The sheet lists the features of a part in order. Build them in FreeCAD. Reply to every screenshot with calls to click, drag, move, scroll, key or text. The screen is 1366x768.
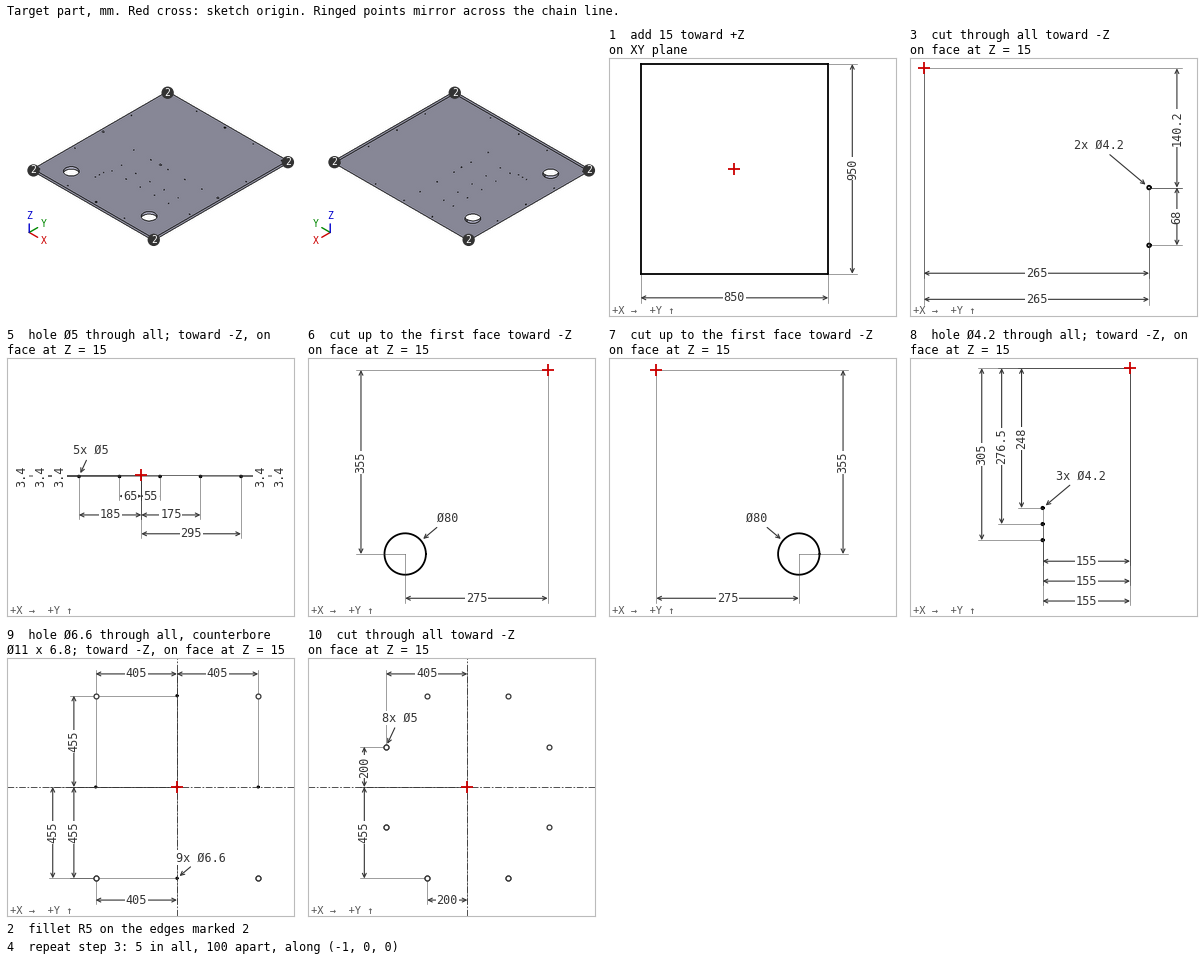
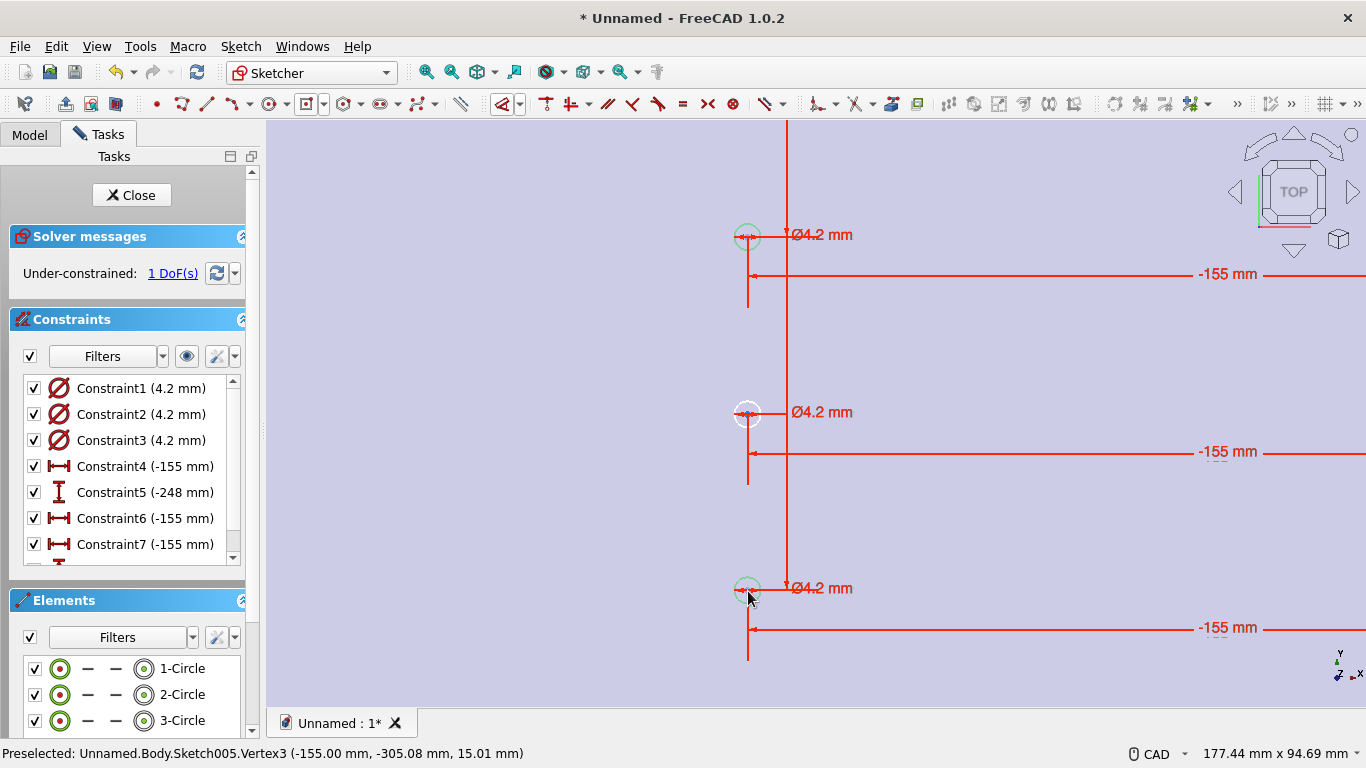
click(748, 414)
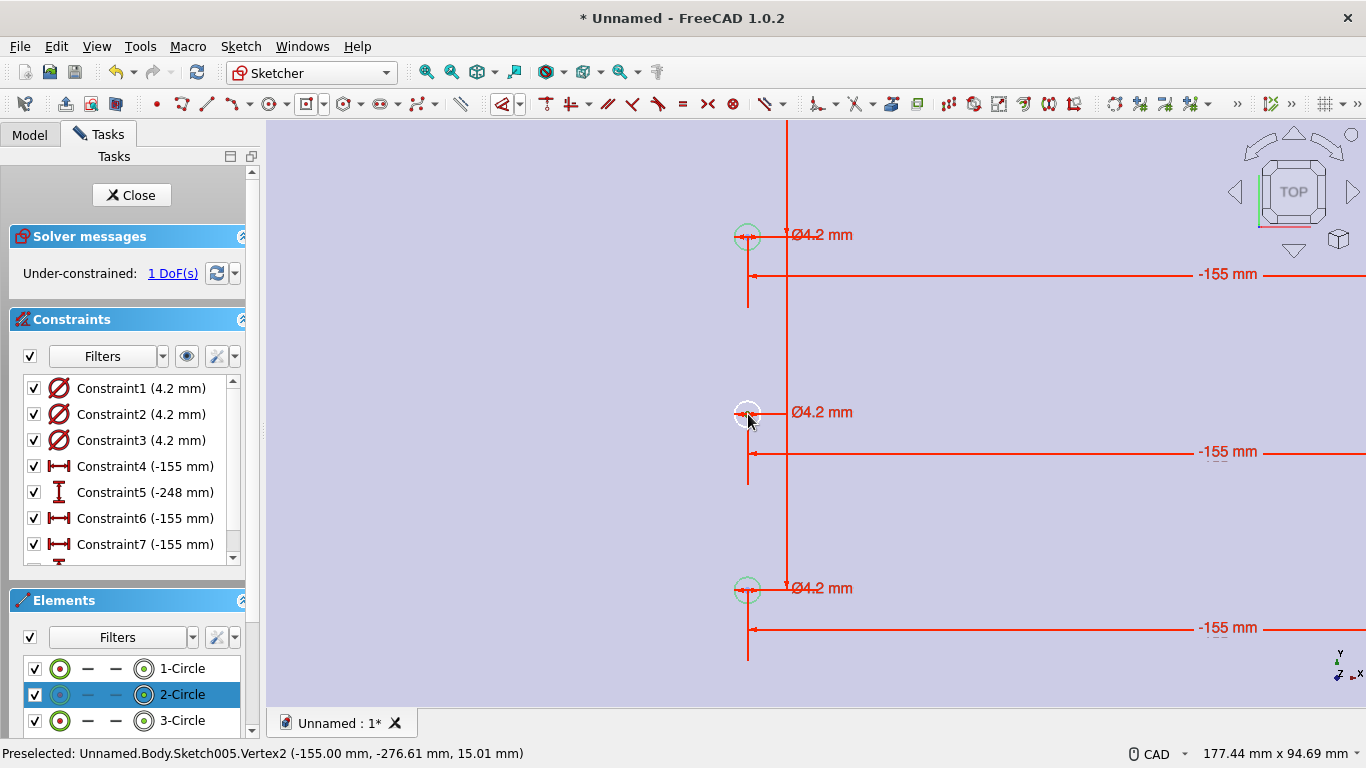
click(520, 104)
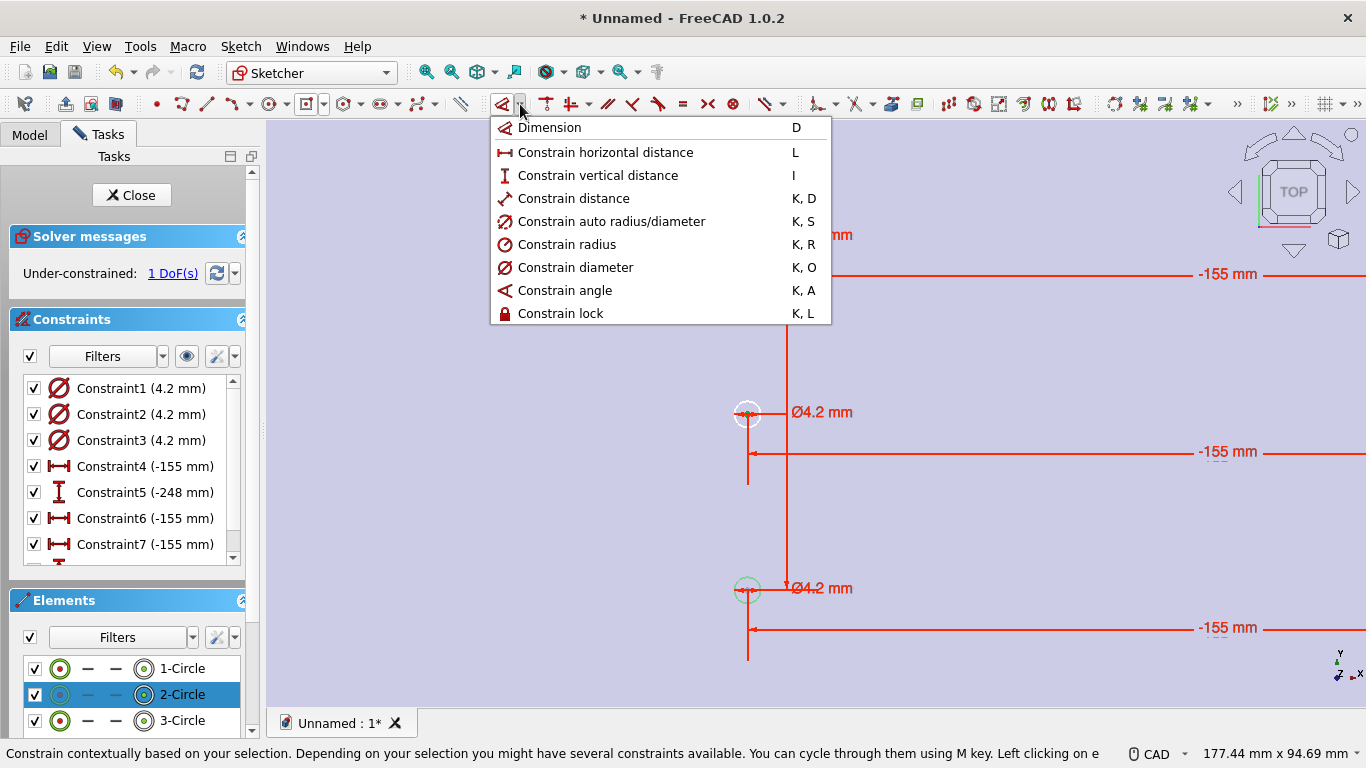
click(661, 176)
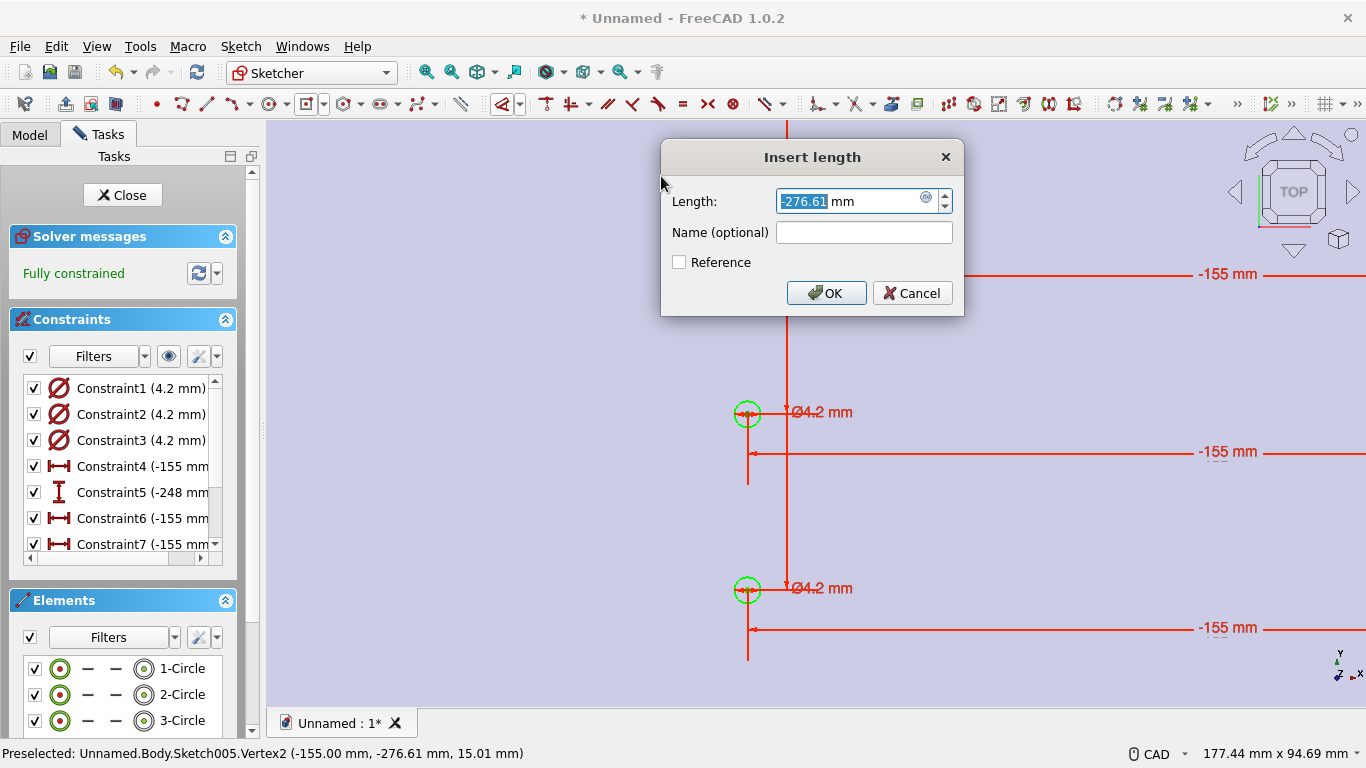
text(-276.5)
key(Return)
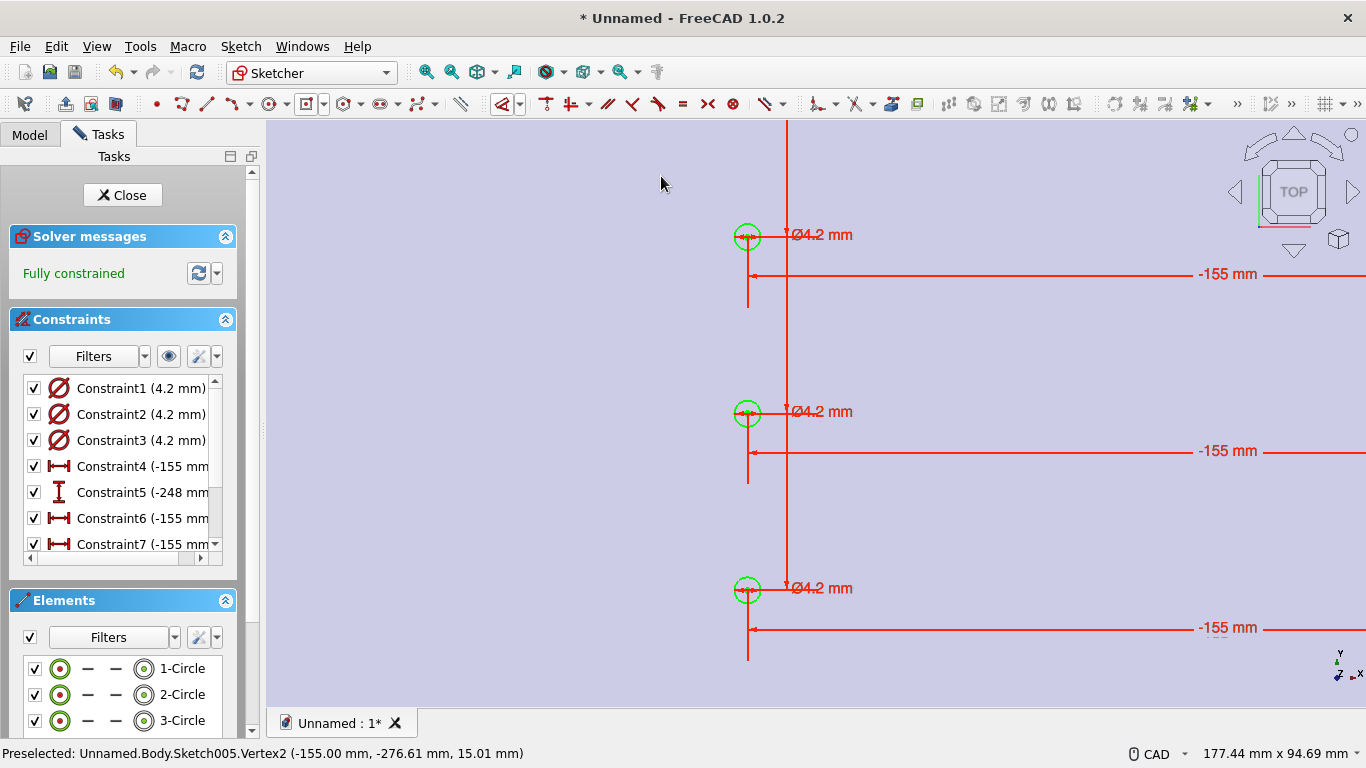
click(123, 195)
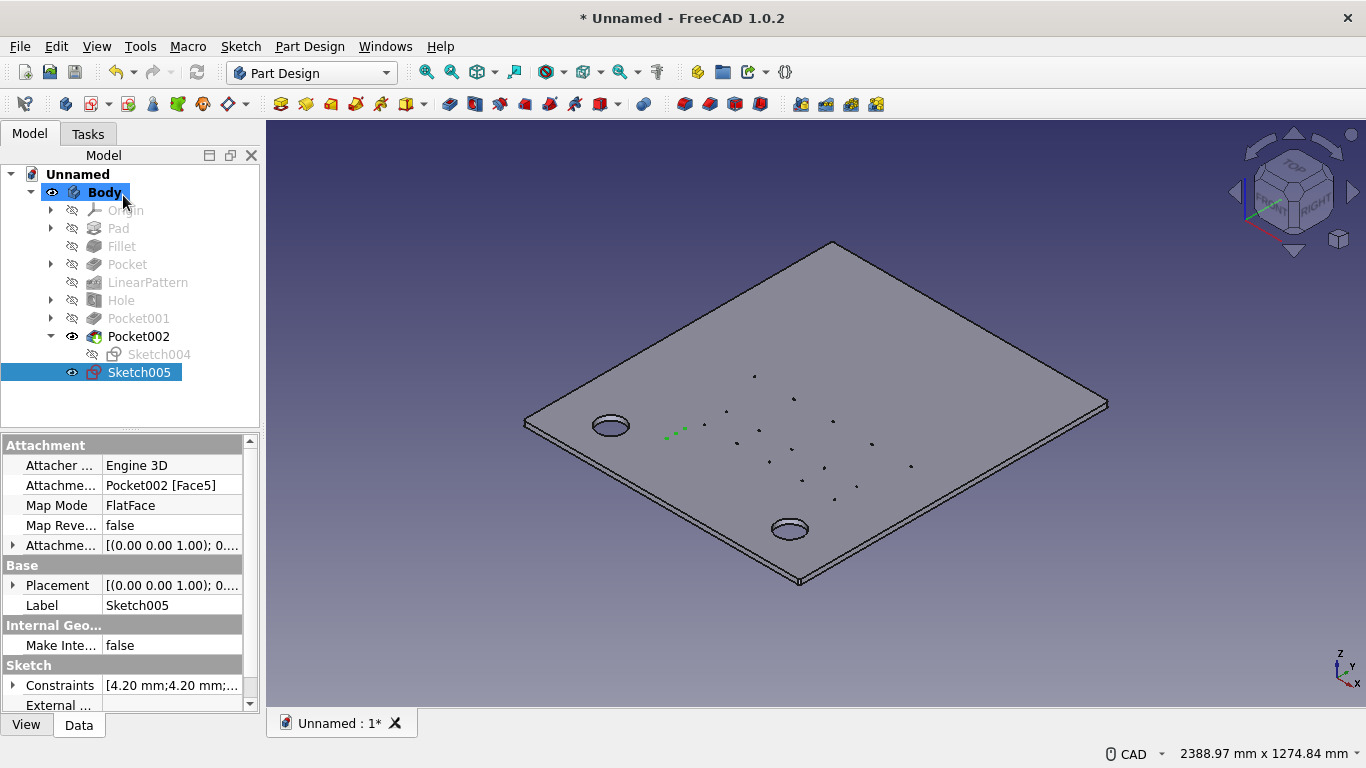
click(475, 104)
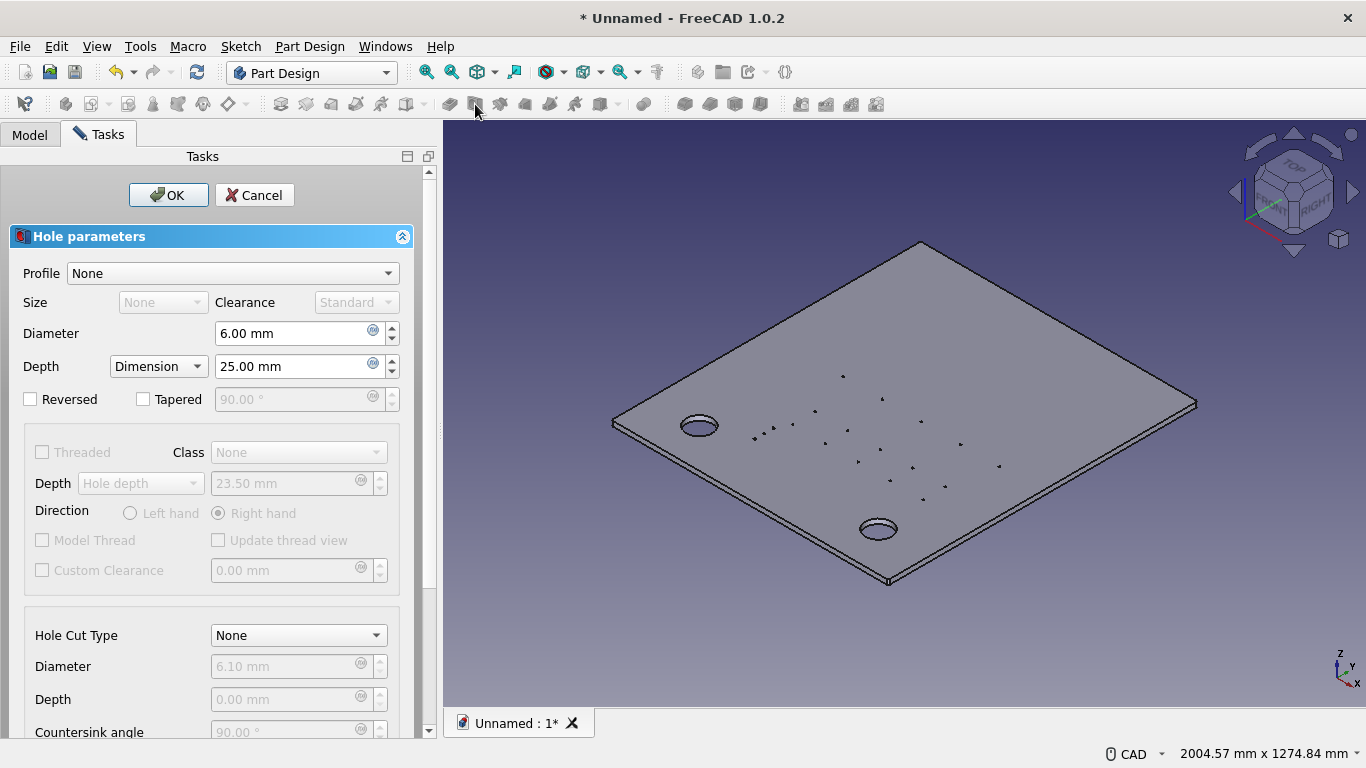
triple_click(300, 334)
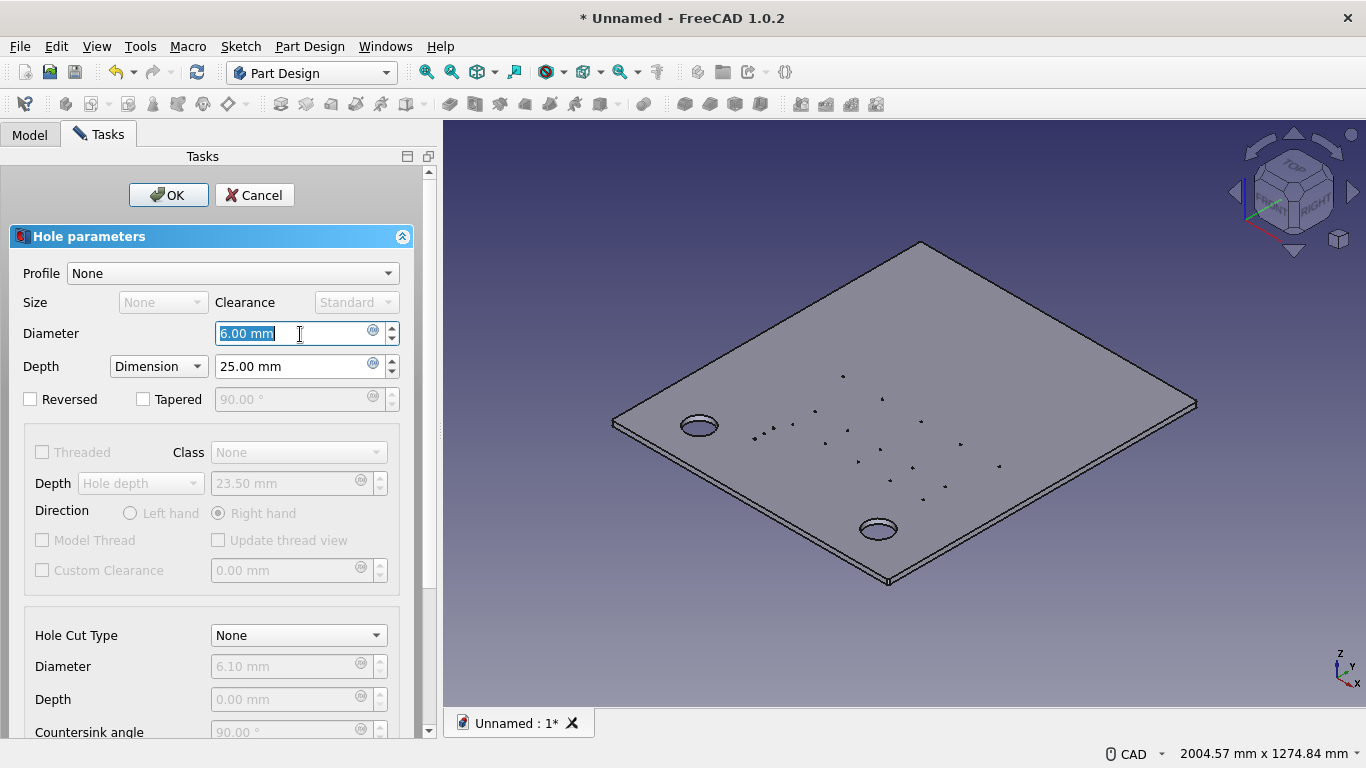
text(4.2)
key(Tab)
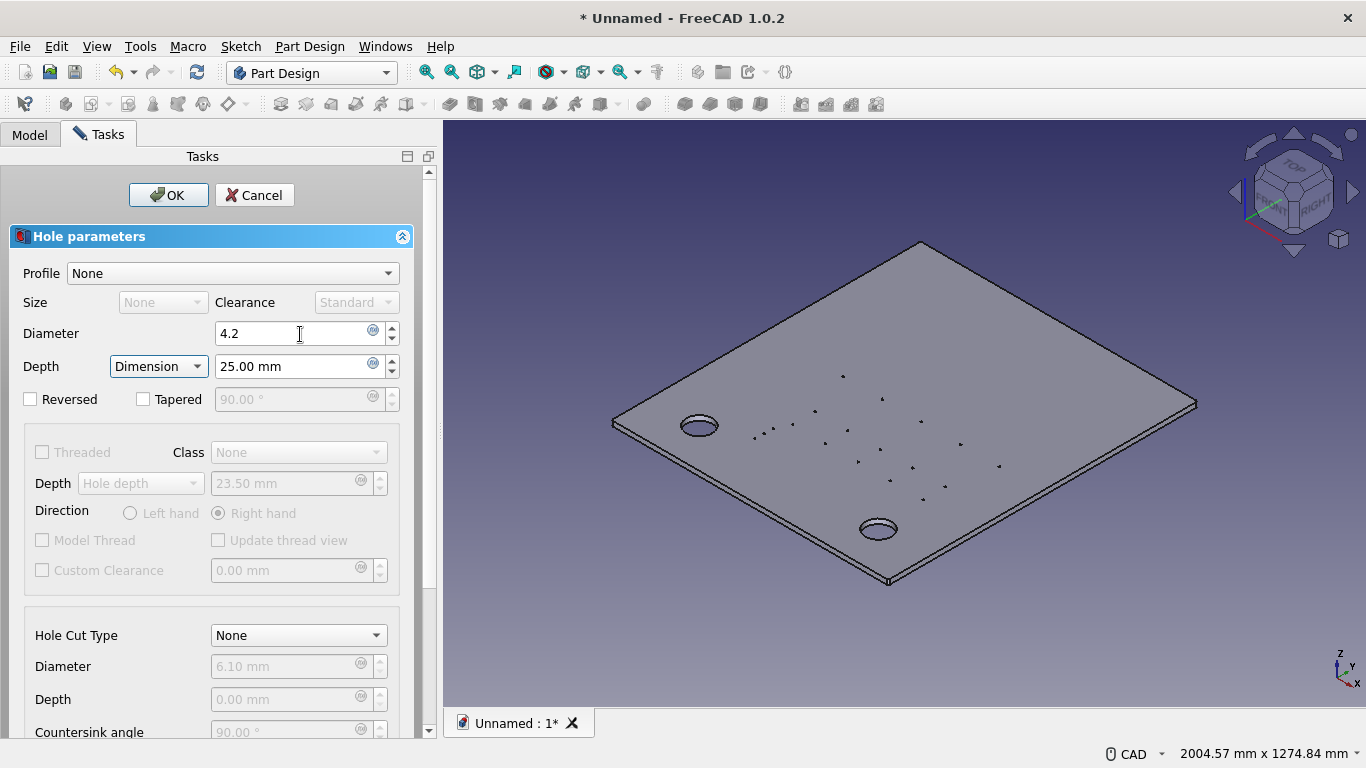
click(160, 366)